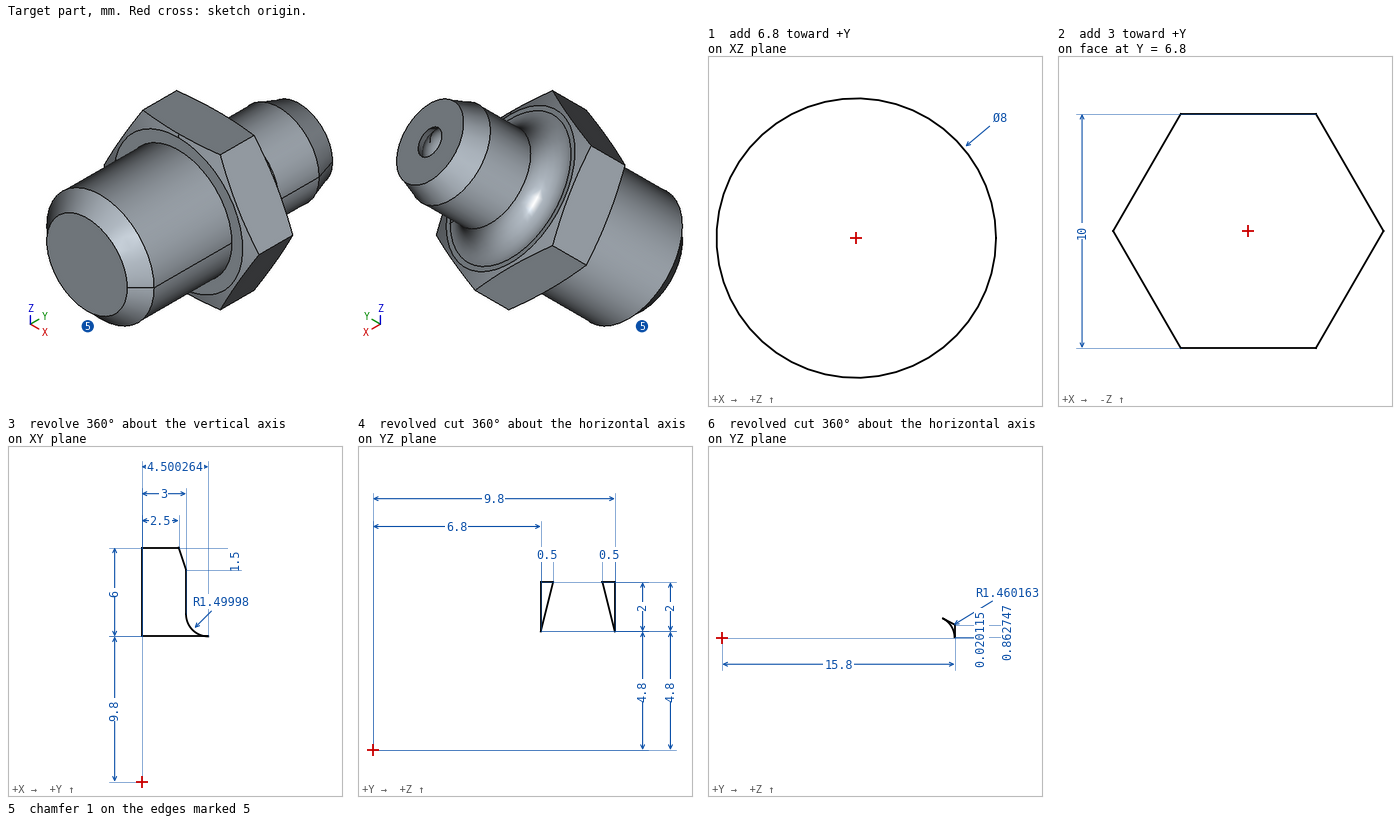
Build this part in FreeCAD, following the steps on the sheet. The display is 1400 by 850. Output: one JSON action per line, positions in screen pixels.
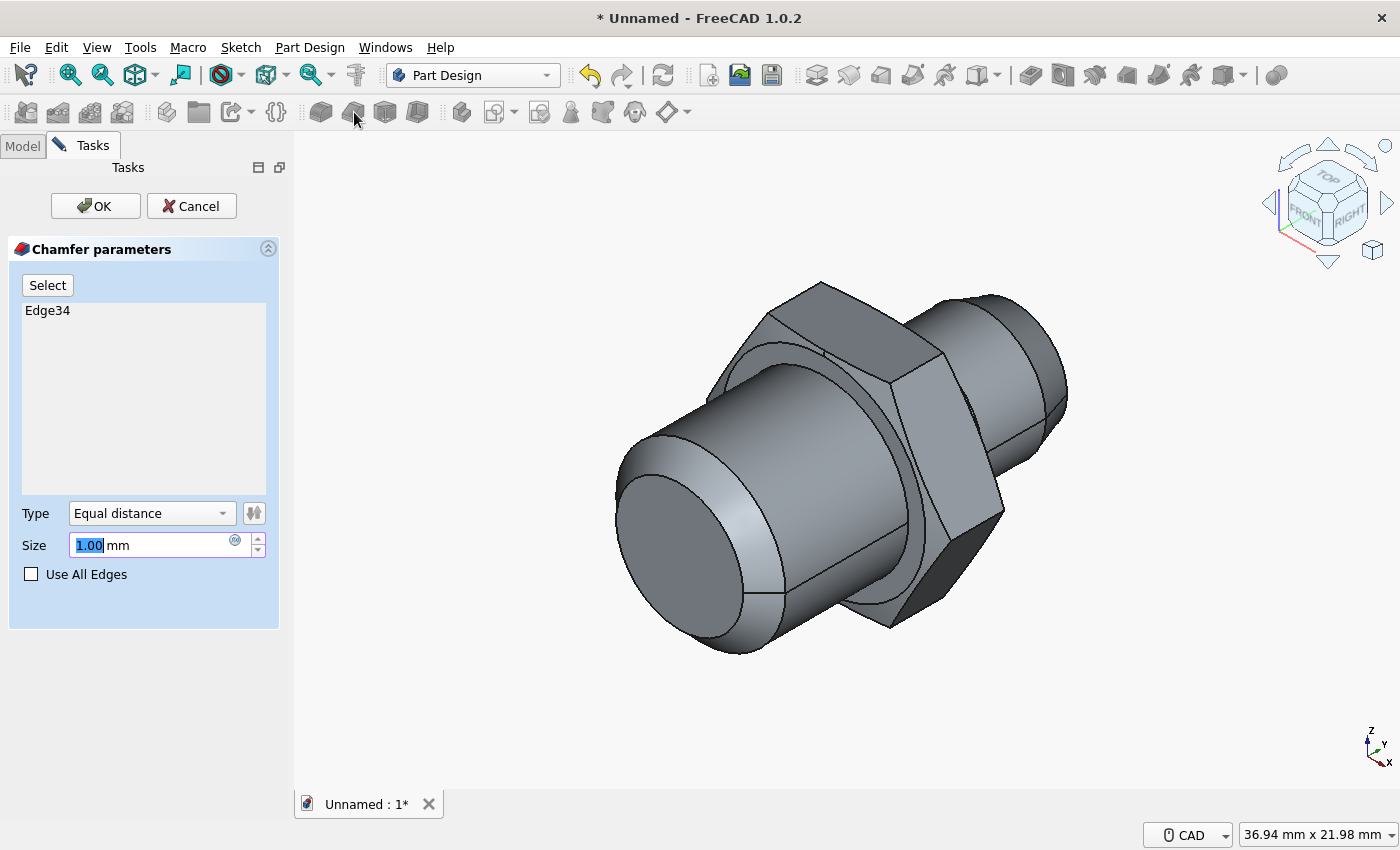
{"action": "type", "text": "1"}
{"action": "key", "text": "Tab"}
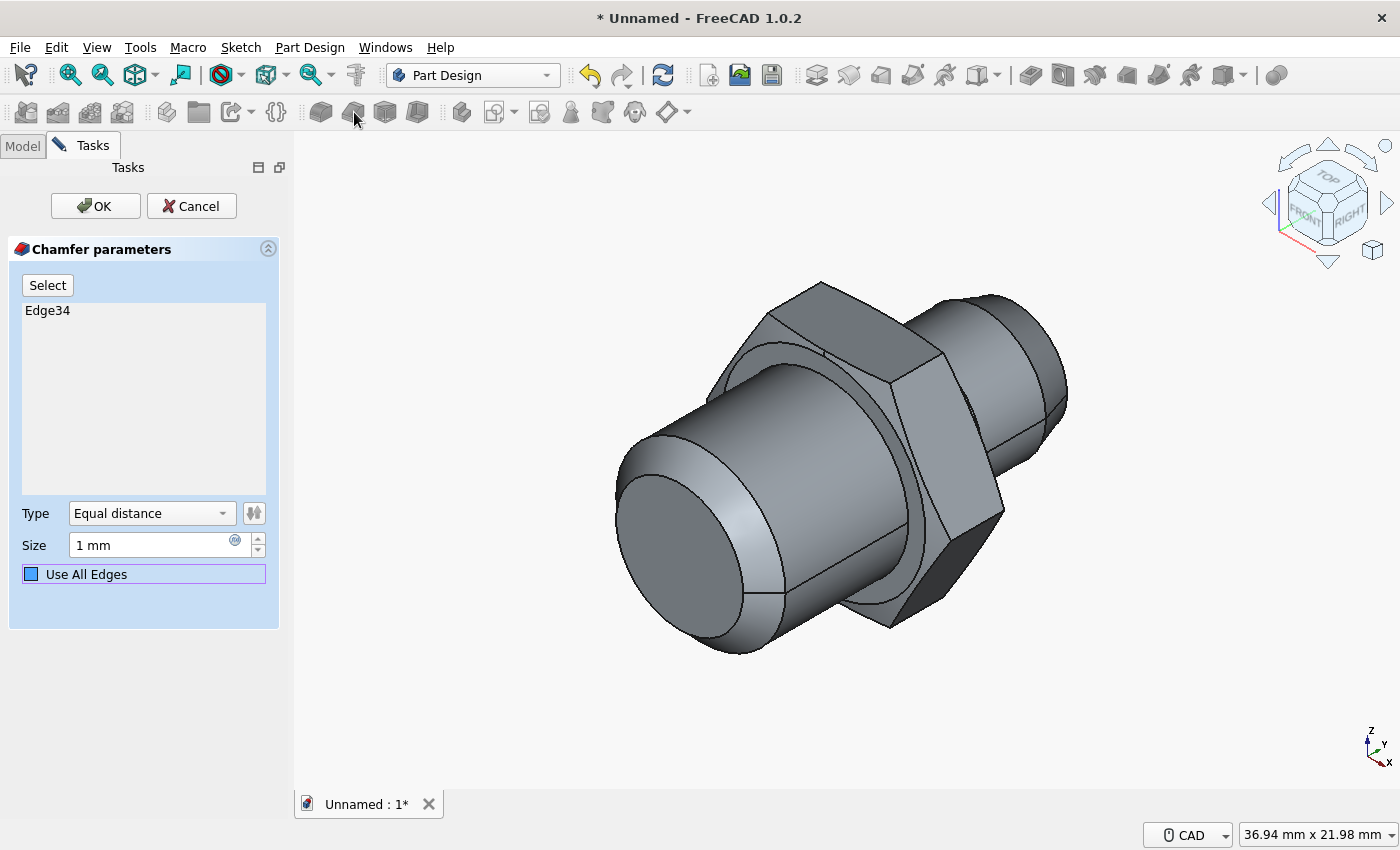
{"action": "left_click", "coordinate": [96, 206]}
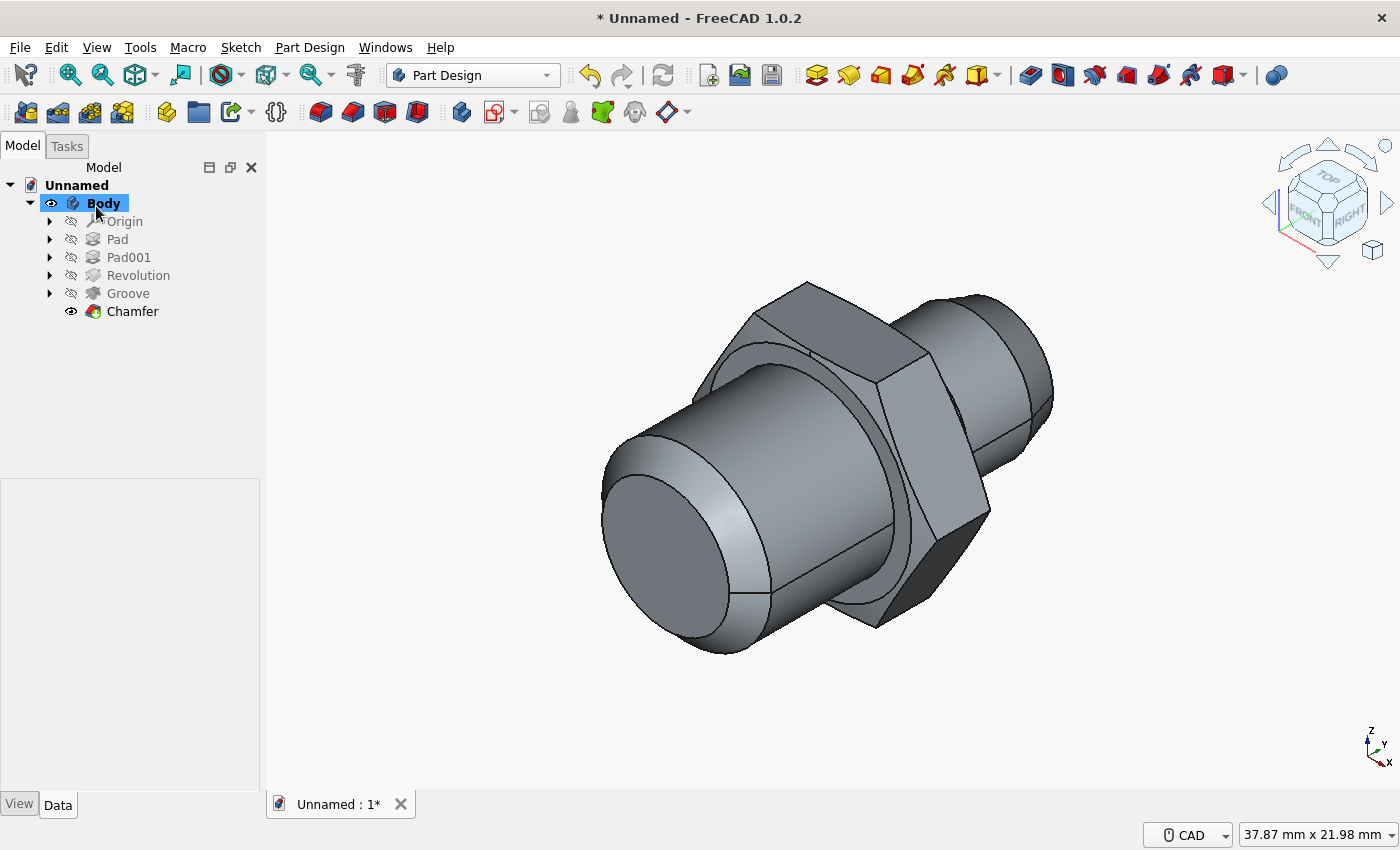
{"action": "left_click", "coordinate": [494, 112]}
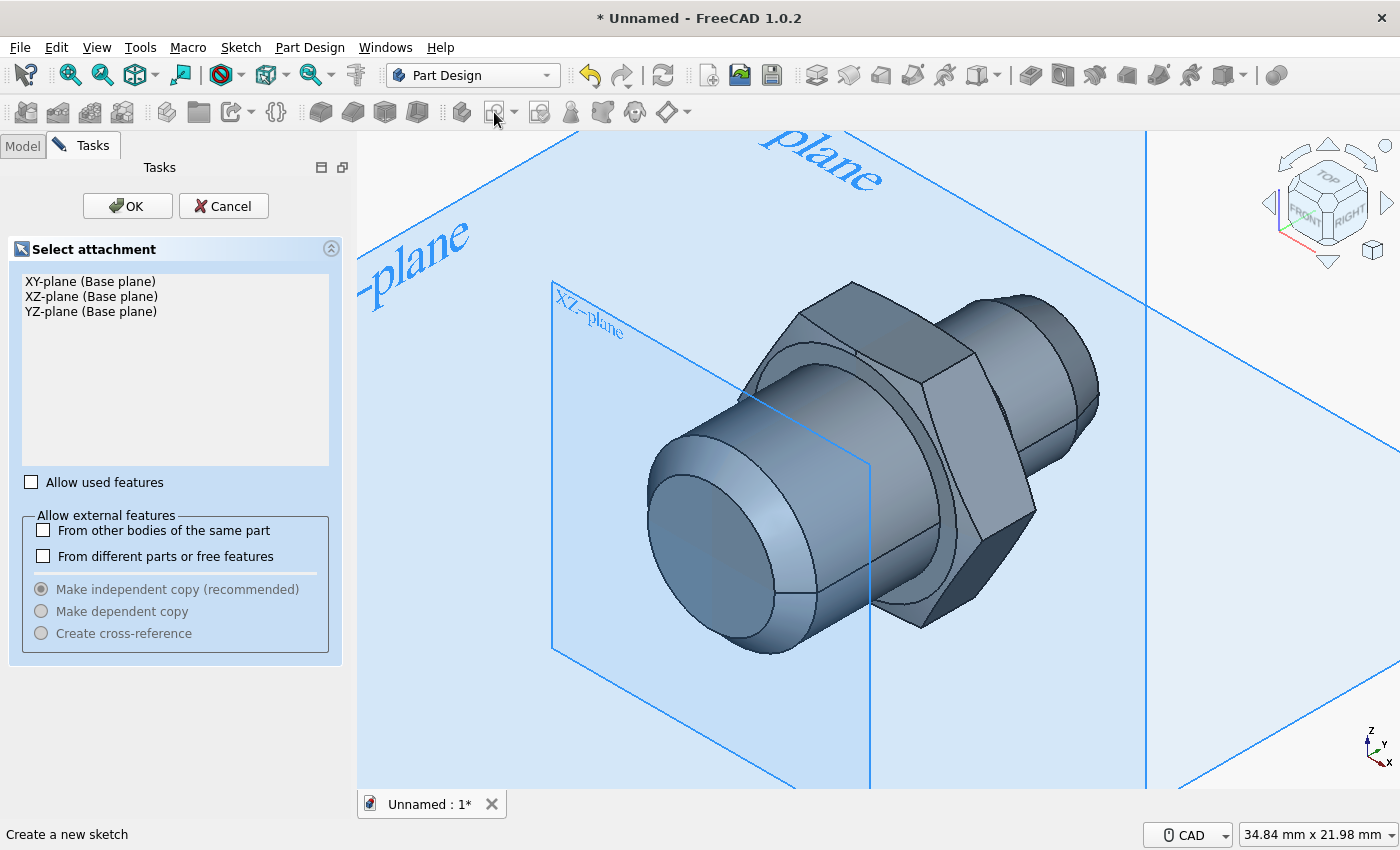
{"action": "left_click", "coordinate": [82, 312]}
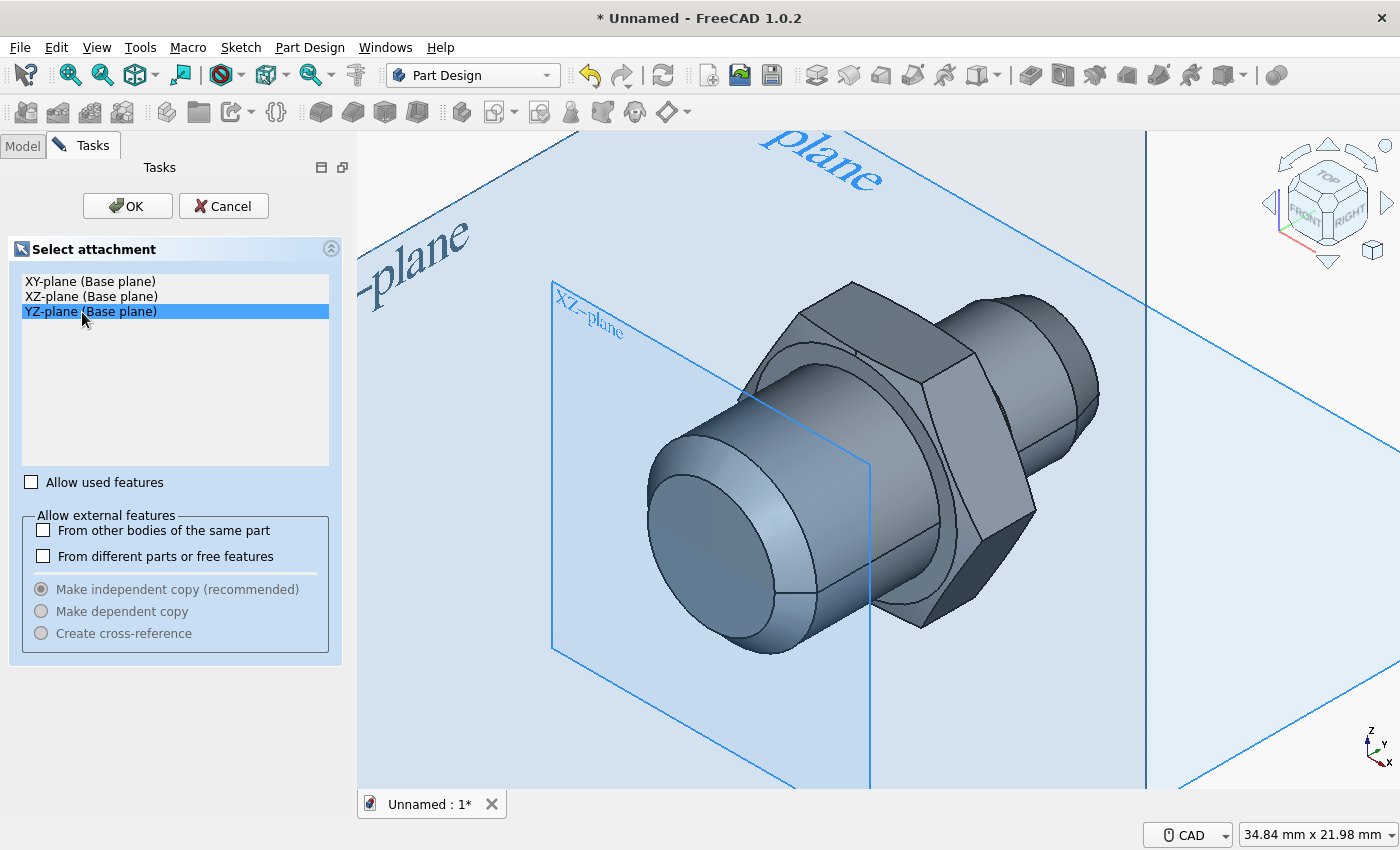
{"action": "left_click", "coordinate": [128, 206]}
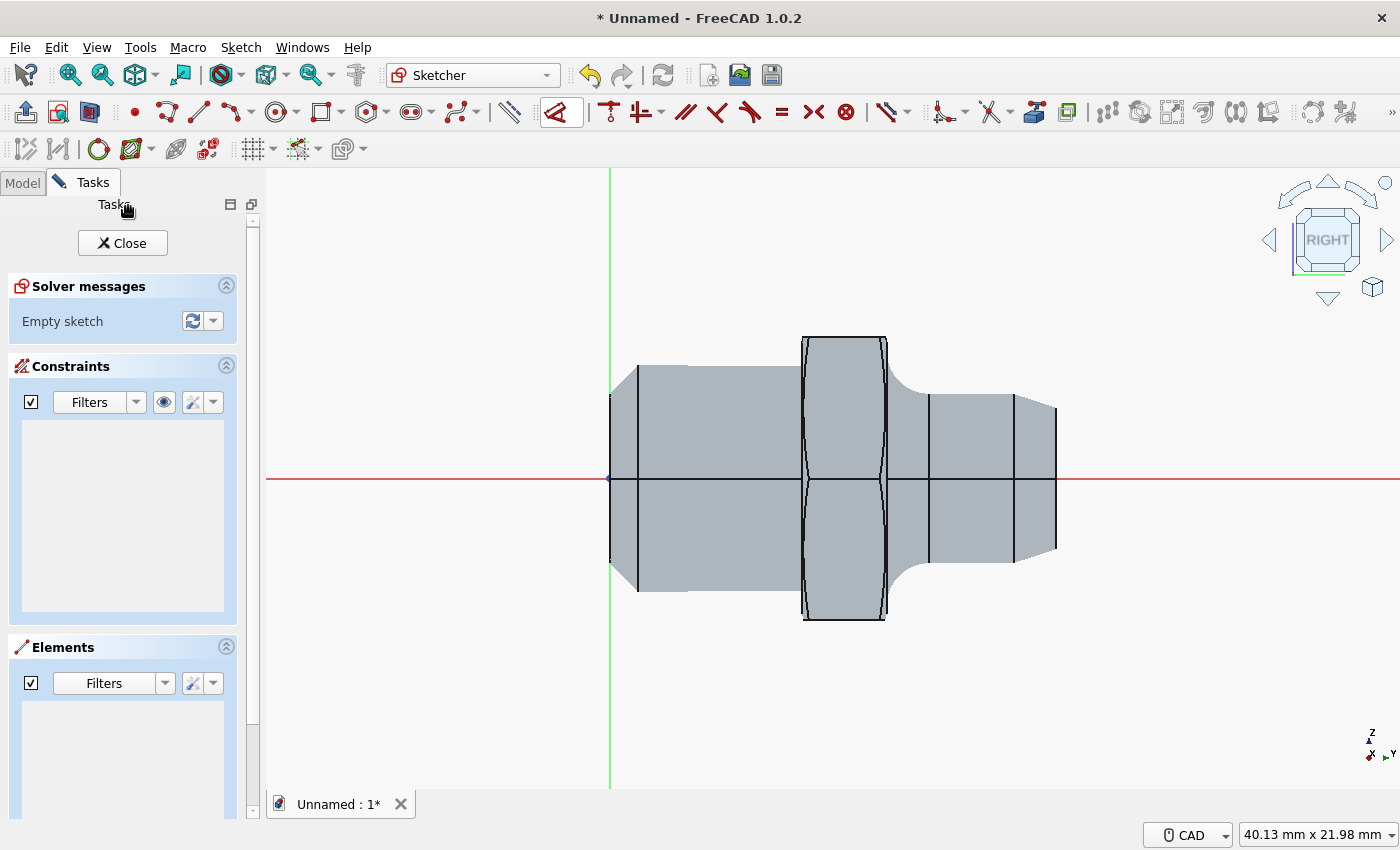
{"action": "left_click", "coordinate": [90, 112]}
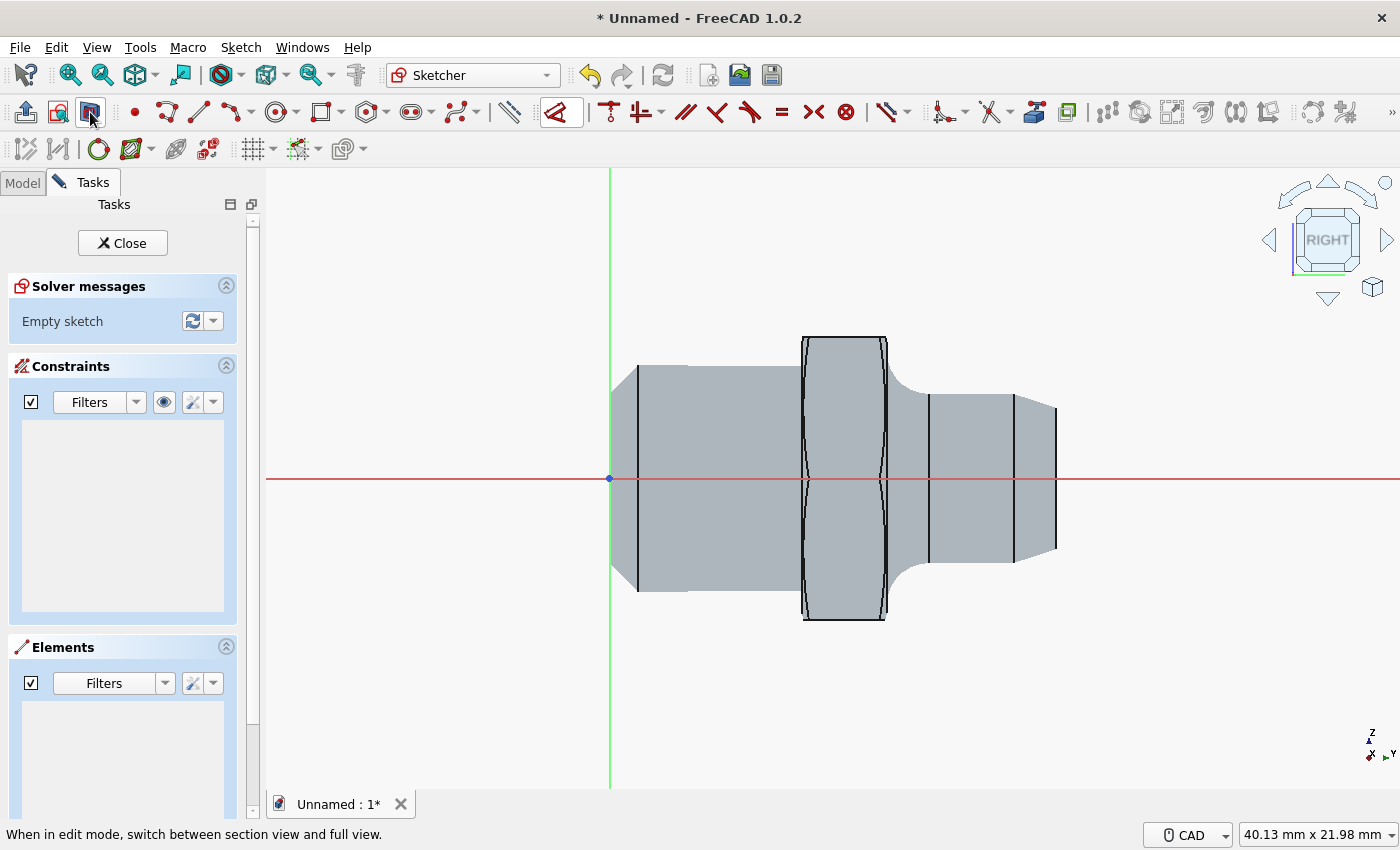
{"action": "scroll", "coordinate": [1073, 458], "scroll_direction": "up", "scroll_amount": 12}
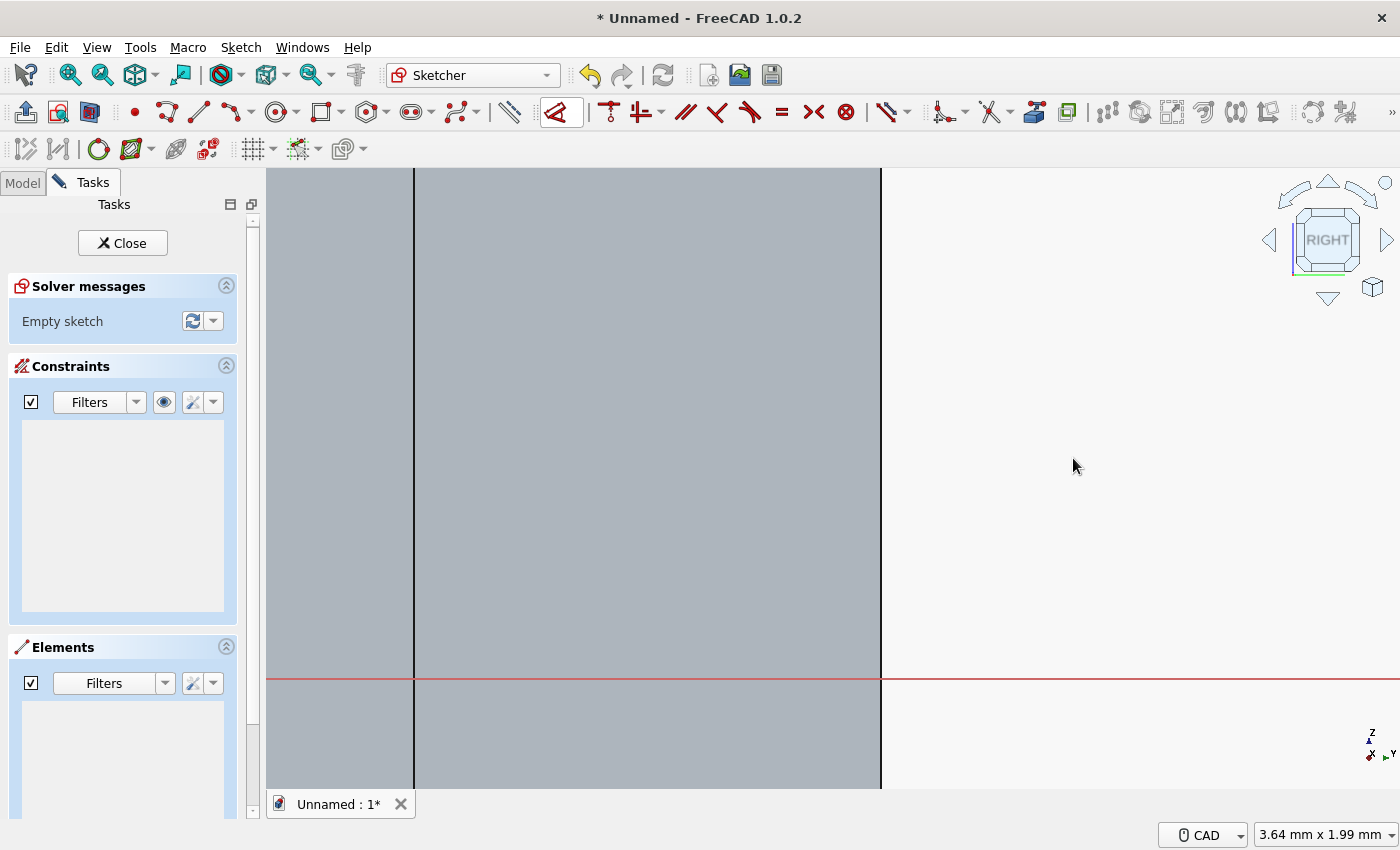
{"action": "left_click", "coordinate": [168, 112]}